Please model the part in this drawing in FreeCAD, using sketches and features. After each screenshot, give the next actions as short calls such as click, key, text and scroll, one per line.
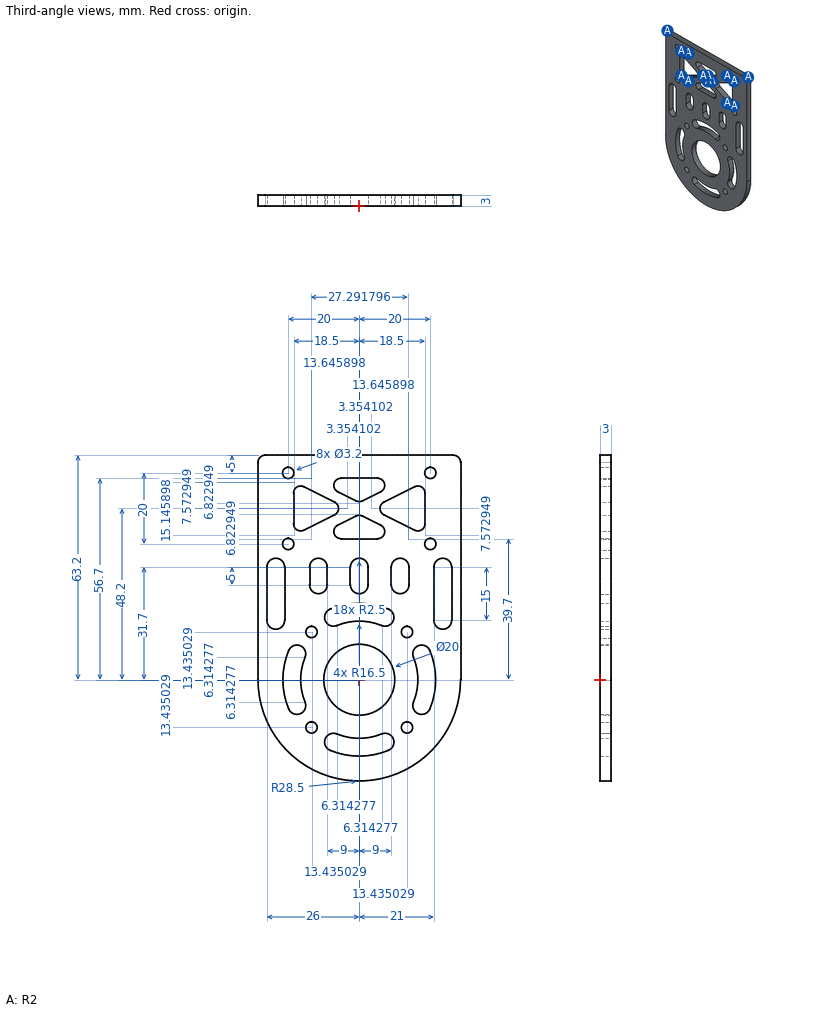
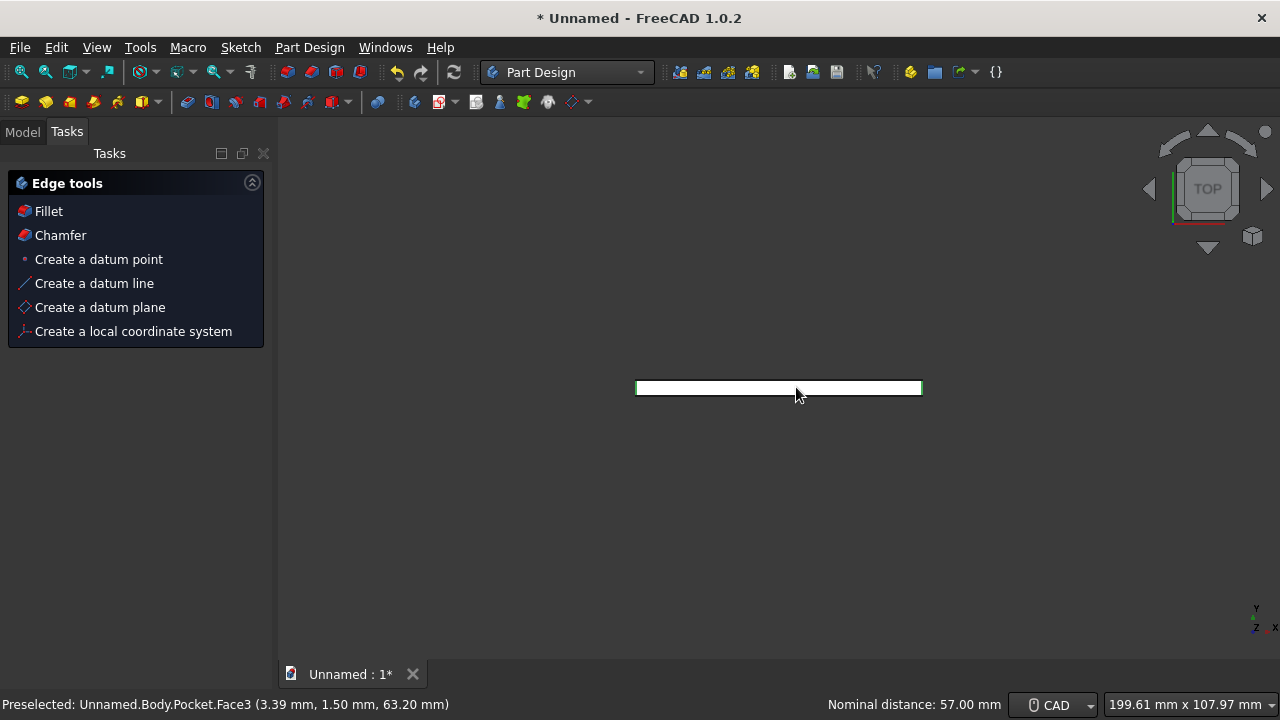
key(1)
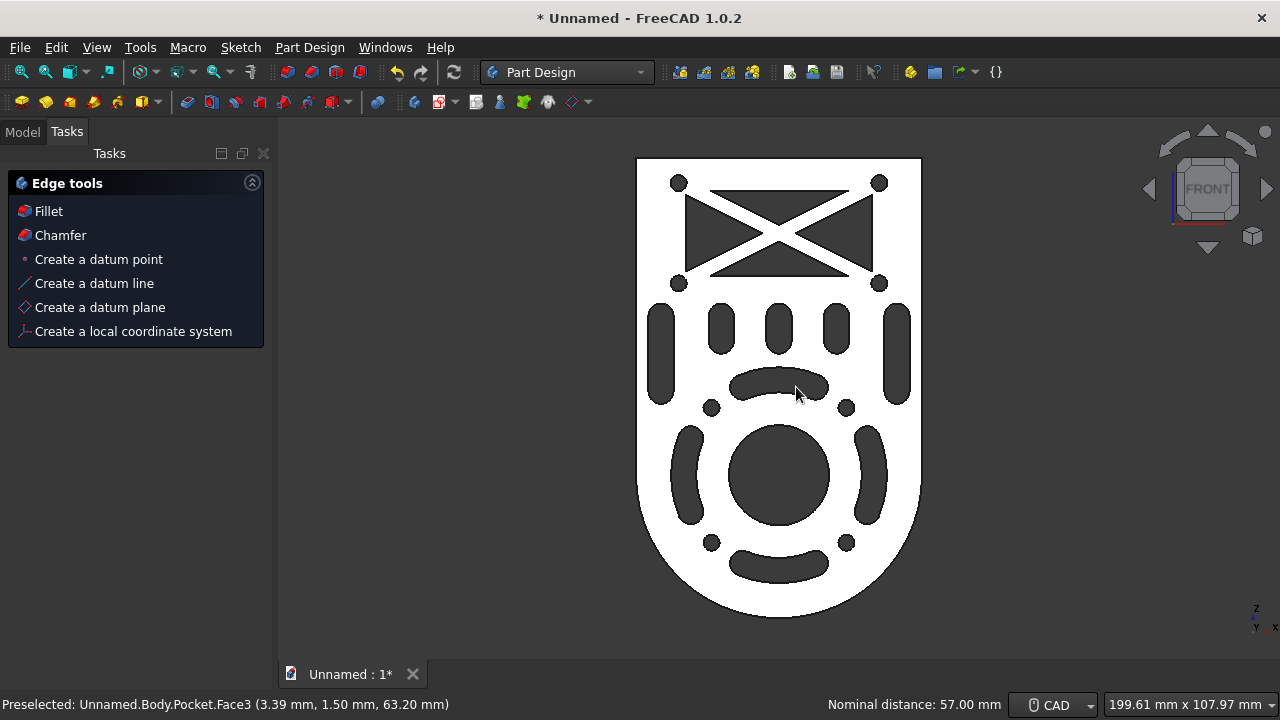
scroll(796, 232, up, 5)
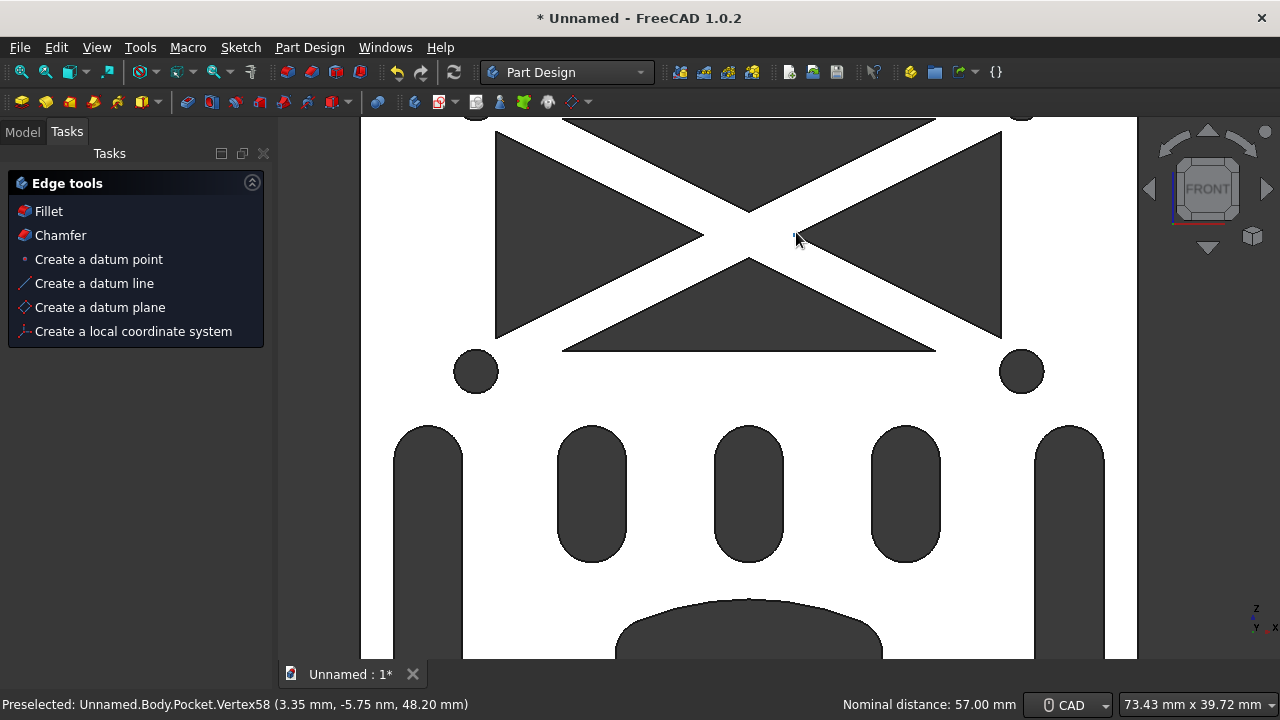
key(v)
key(f)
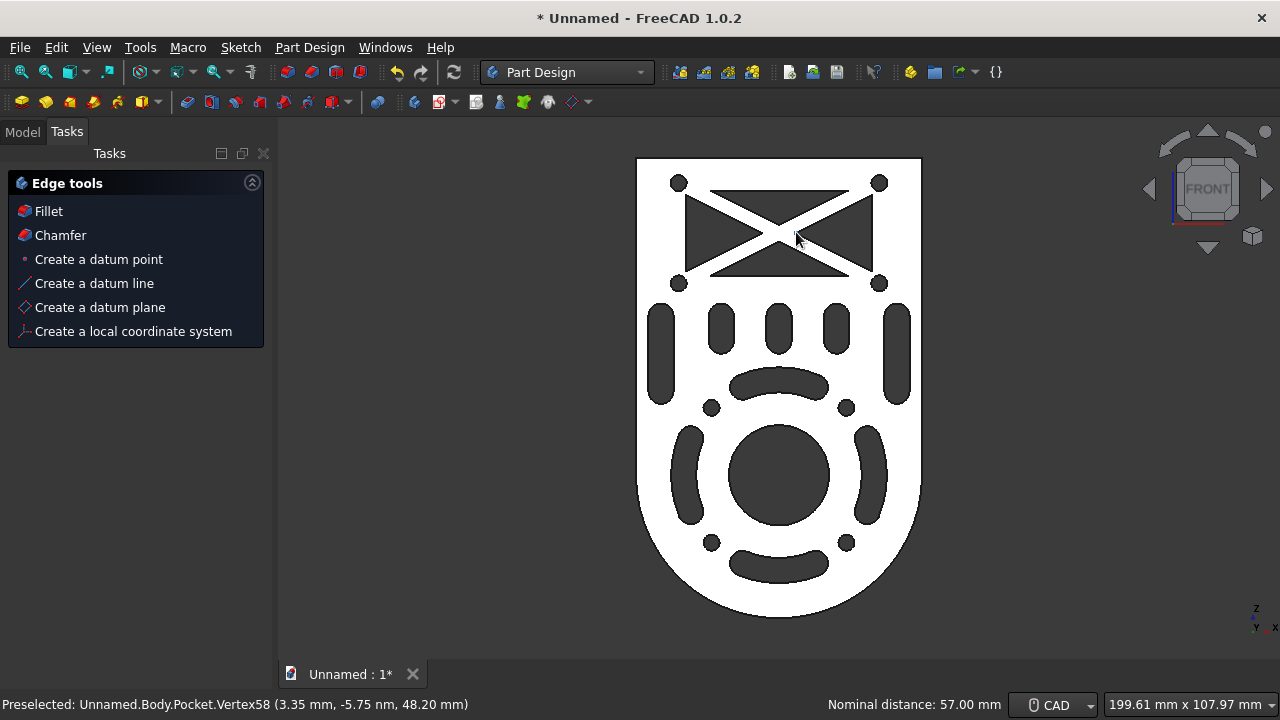
key(3)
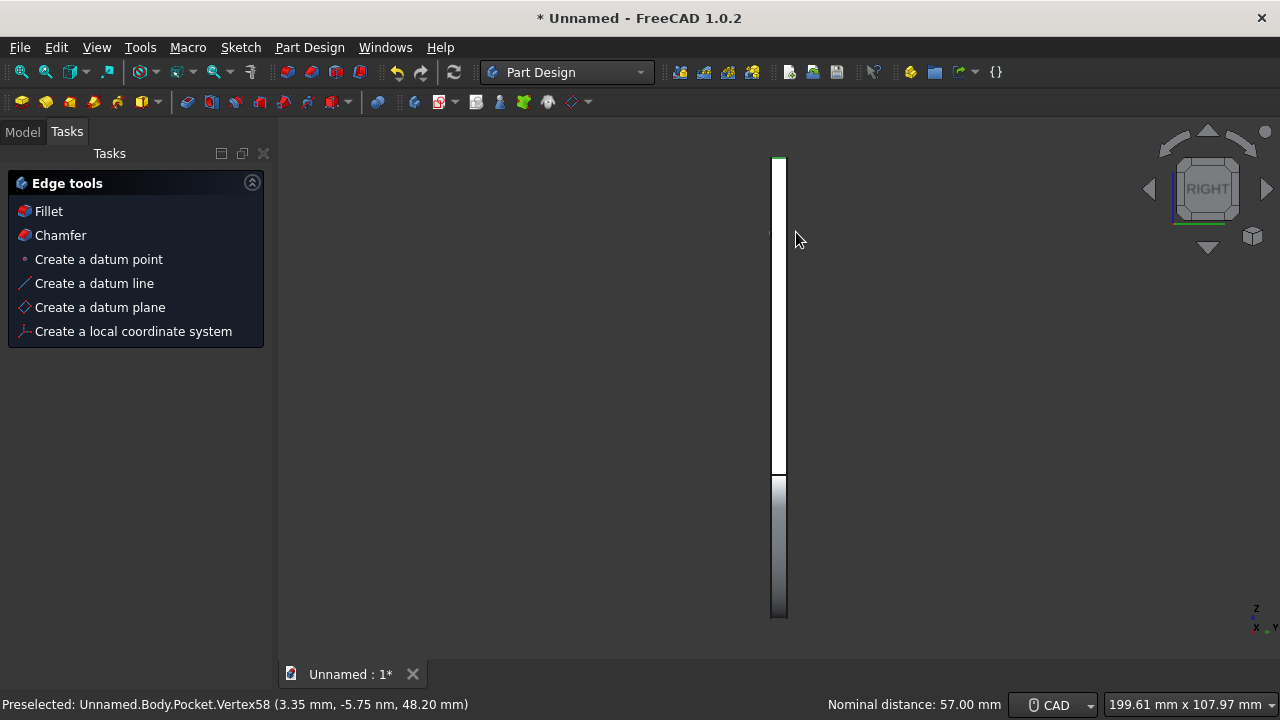
scroll(779, 232, up, 5)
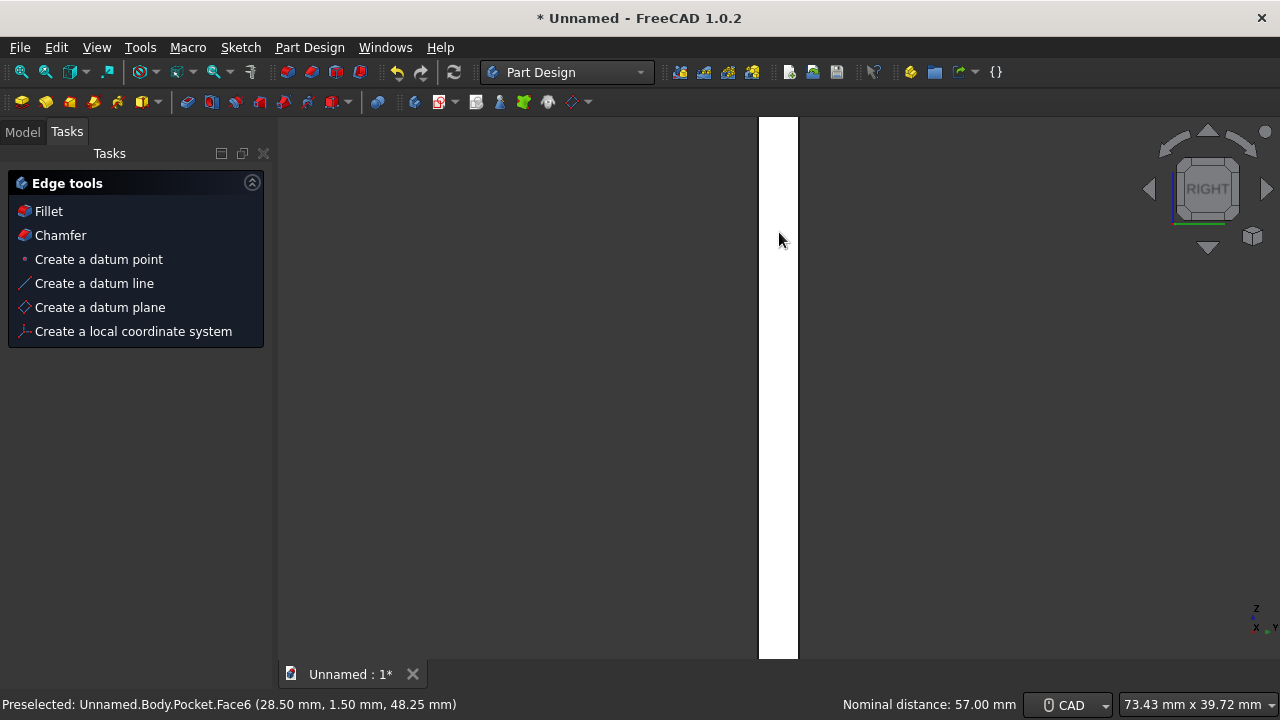
key(v)
key(f)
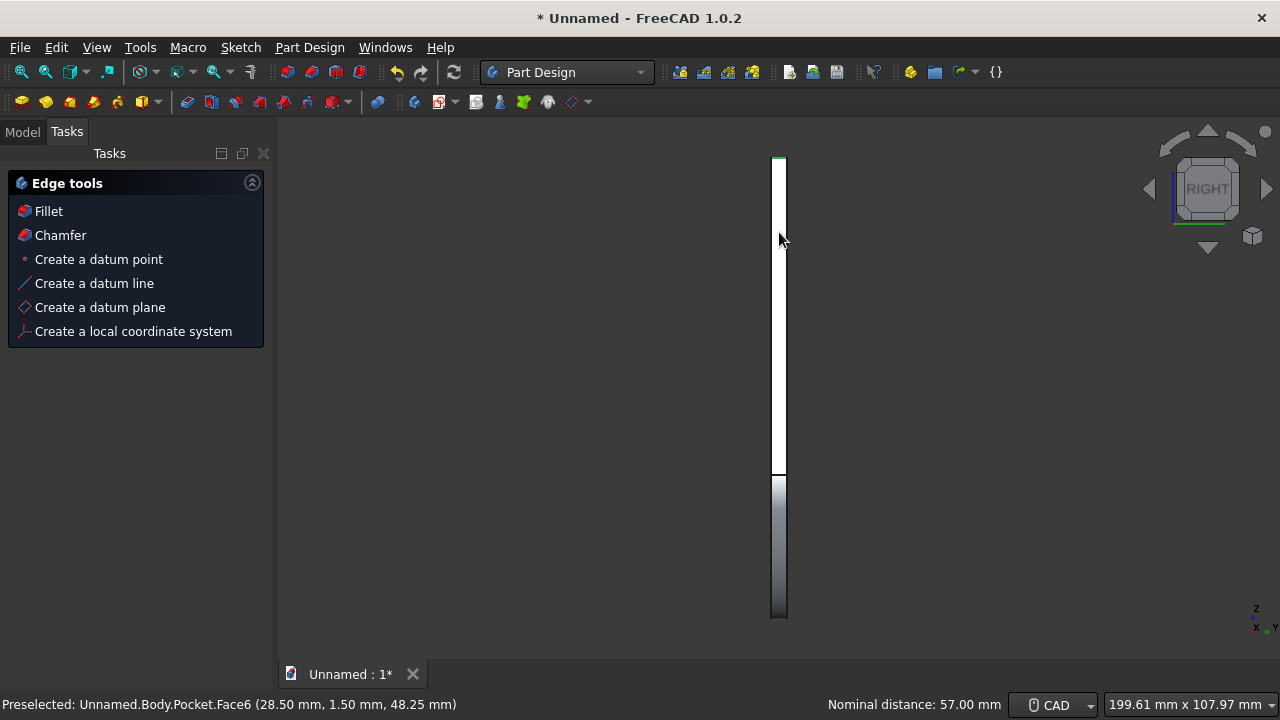
key(5)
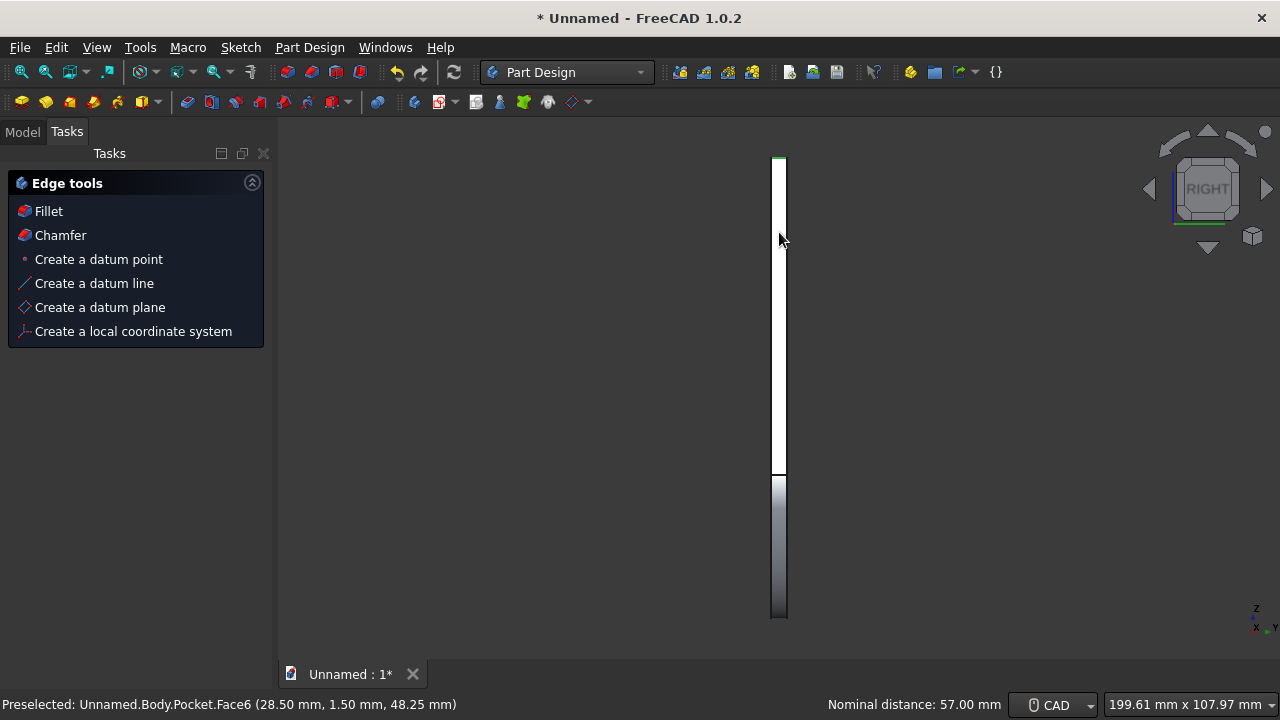
click(22, 72)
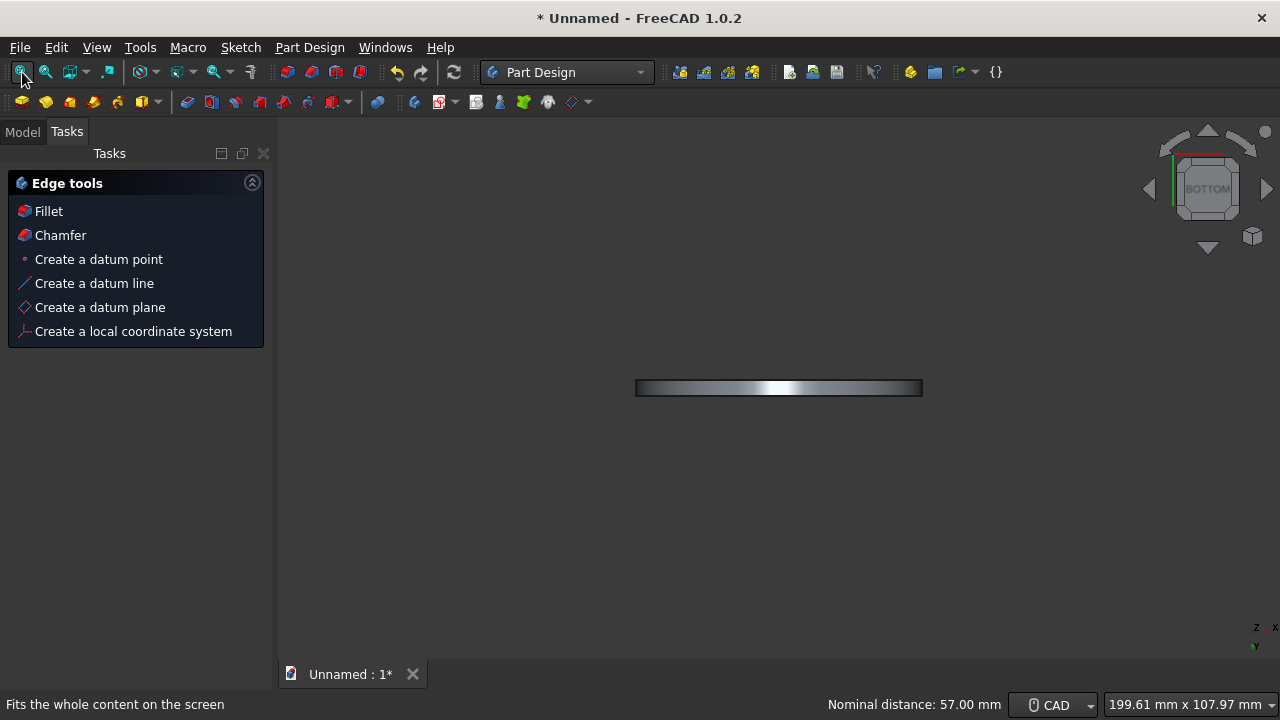
scroll(796, 387, up, 5)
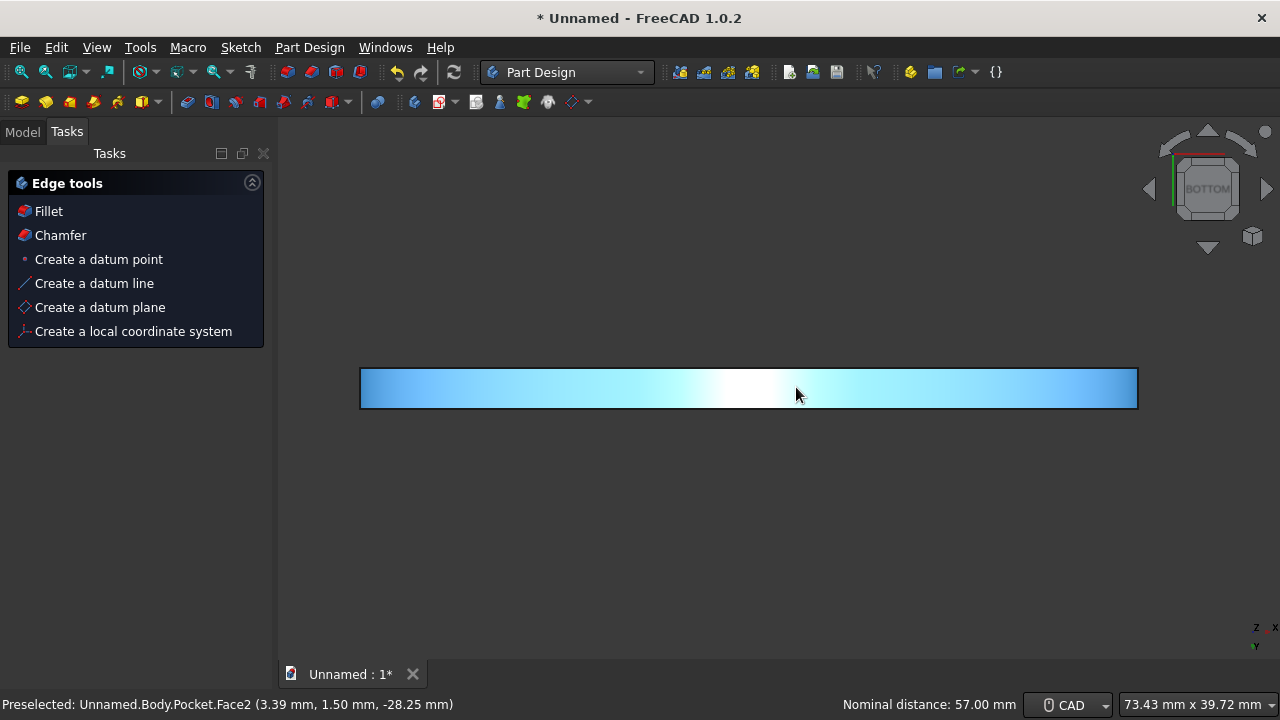
key(v)
key(f)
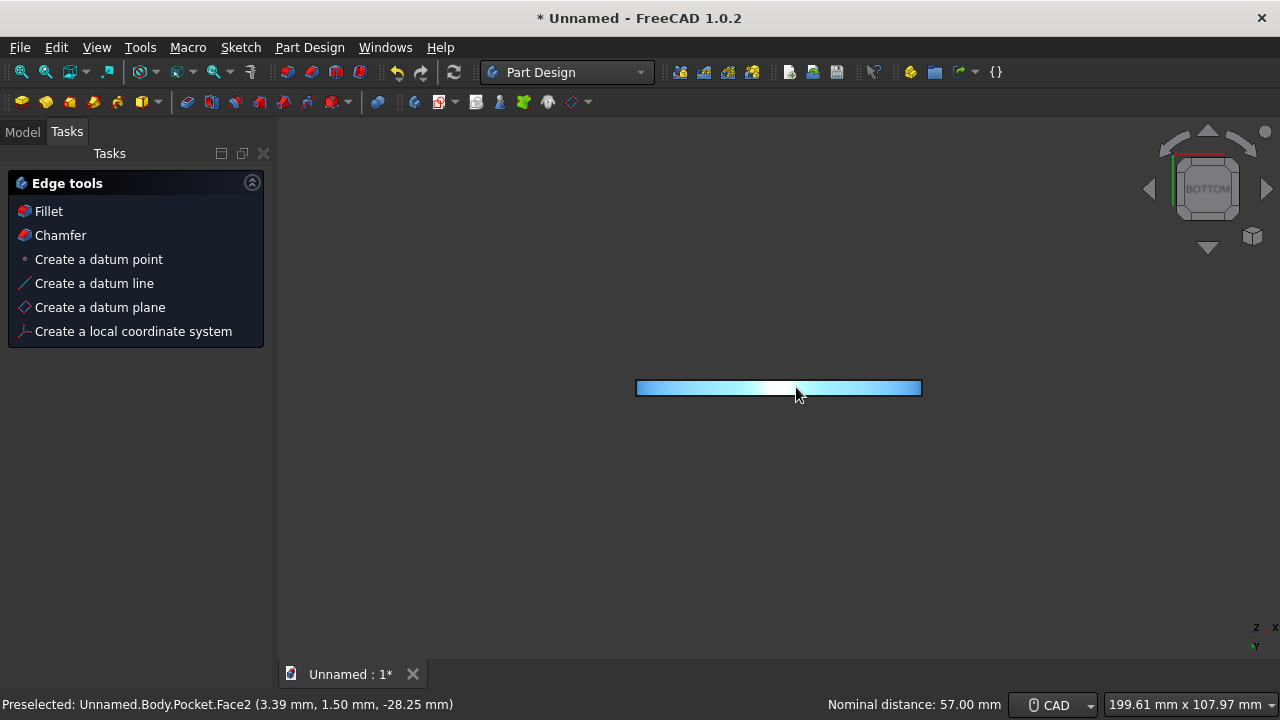
key(4)